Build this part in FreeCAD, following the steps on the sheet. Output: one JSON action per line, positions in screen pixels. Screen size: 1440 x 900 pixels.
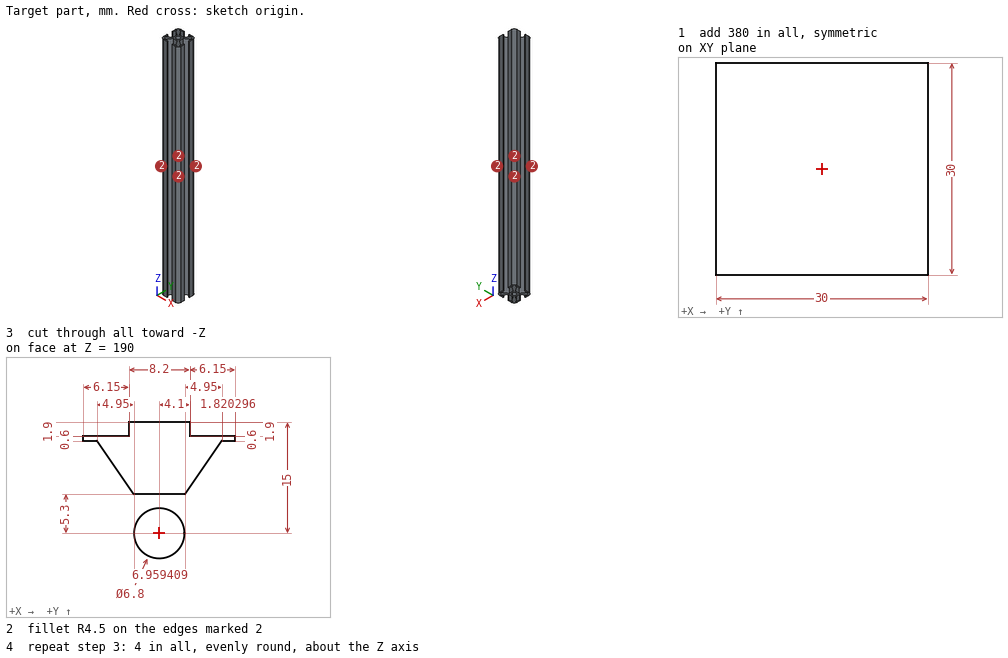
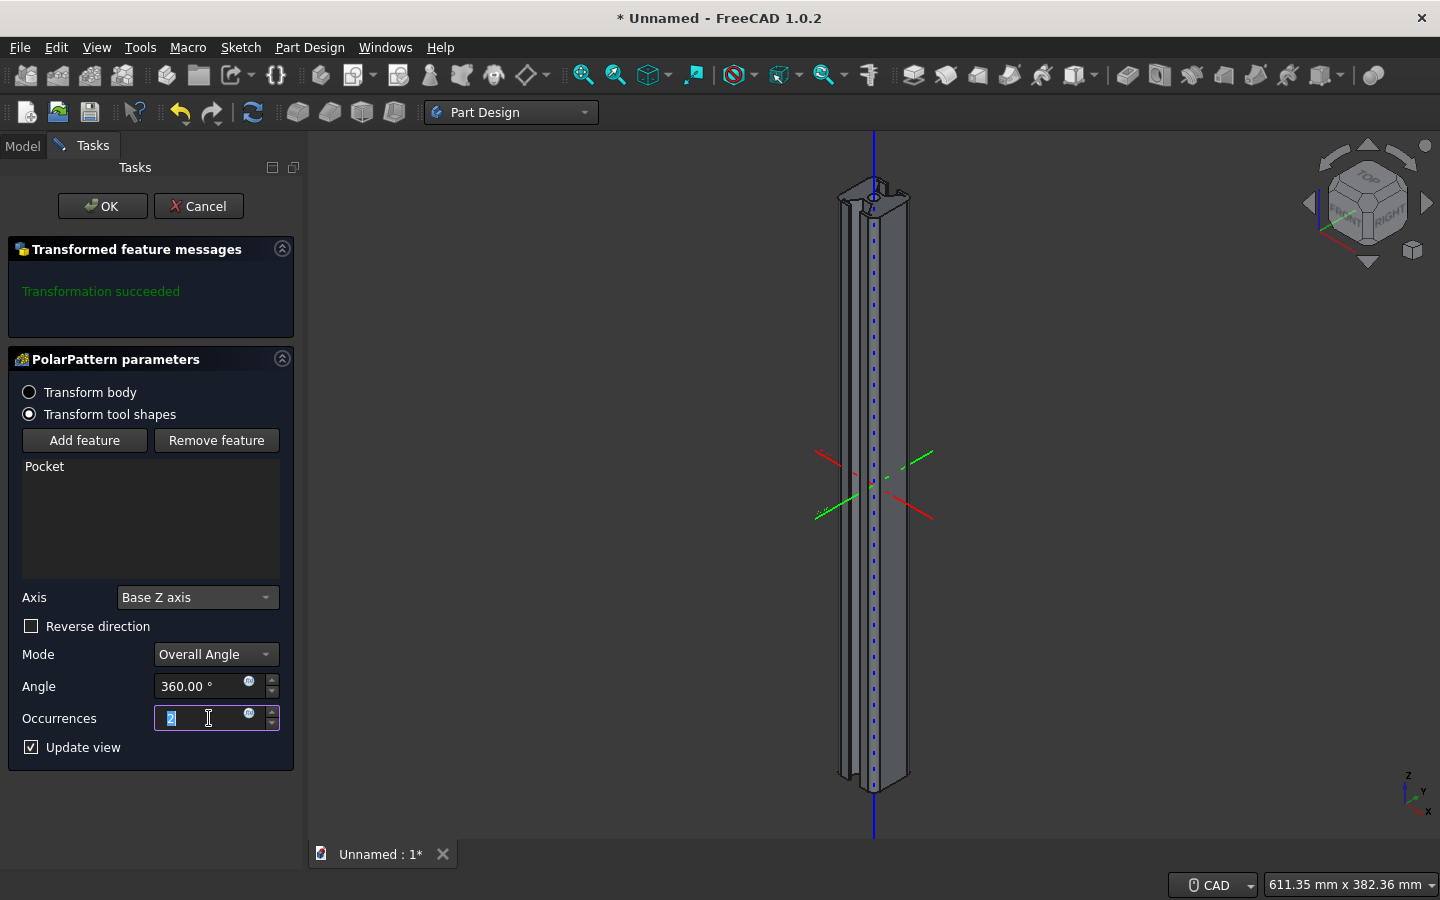
{"action": "type", "text": "4"}
{"action": "key", "text": "Tab"}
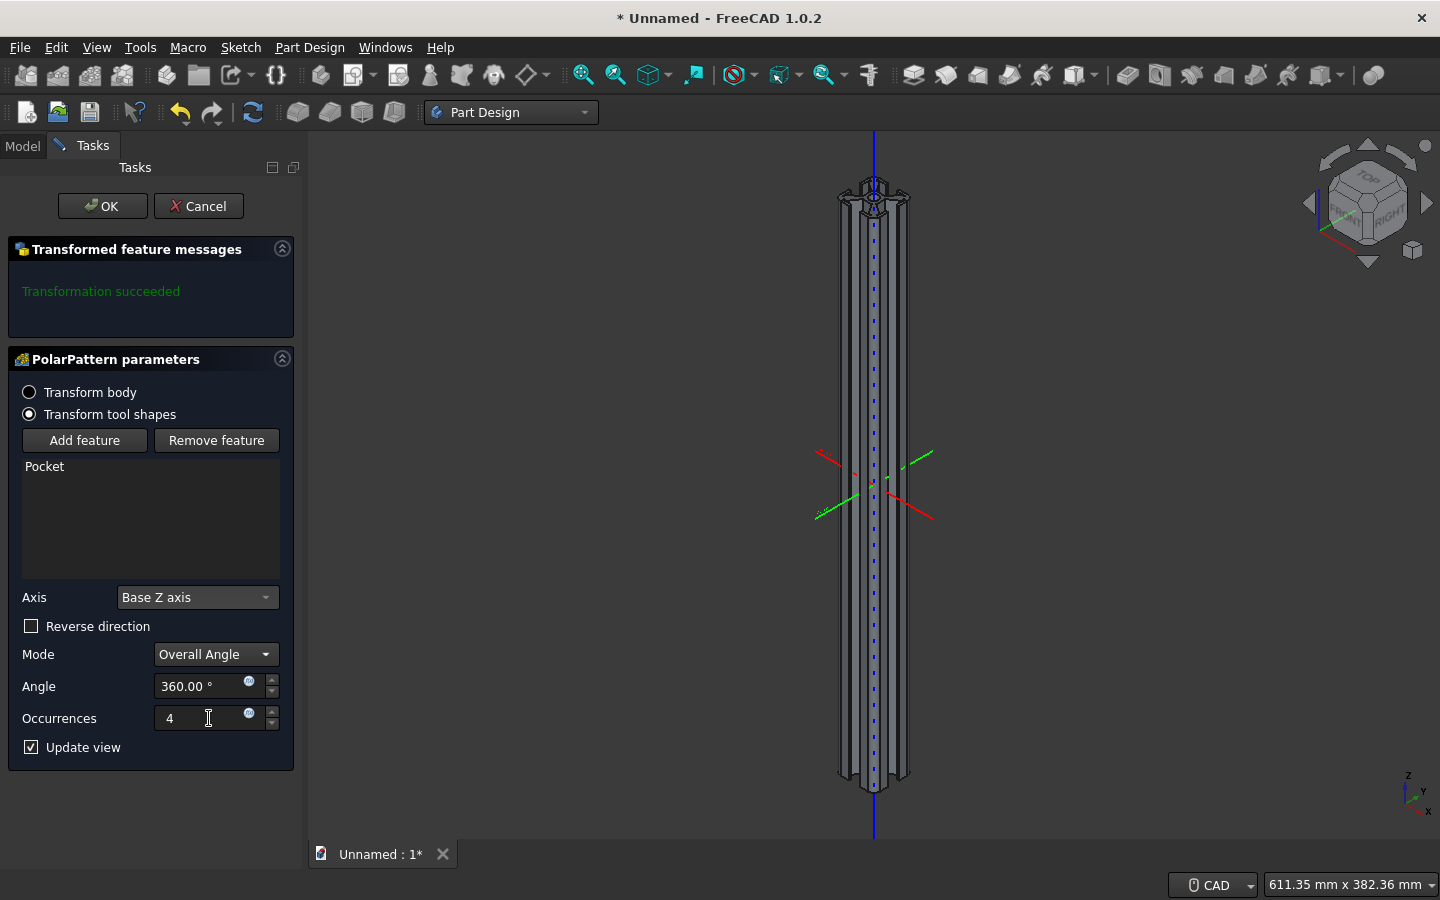
{"action": "left_click", "coordinate": [103, 206]}